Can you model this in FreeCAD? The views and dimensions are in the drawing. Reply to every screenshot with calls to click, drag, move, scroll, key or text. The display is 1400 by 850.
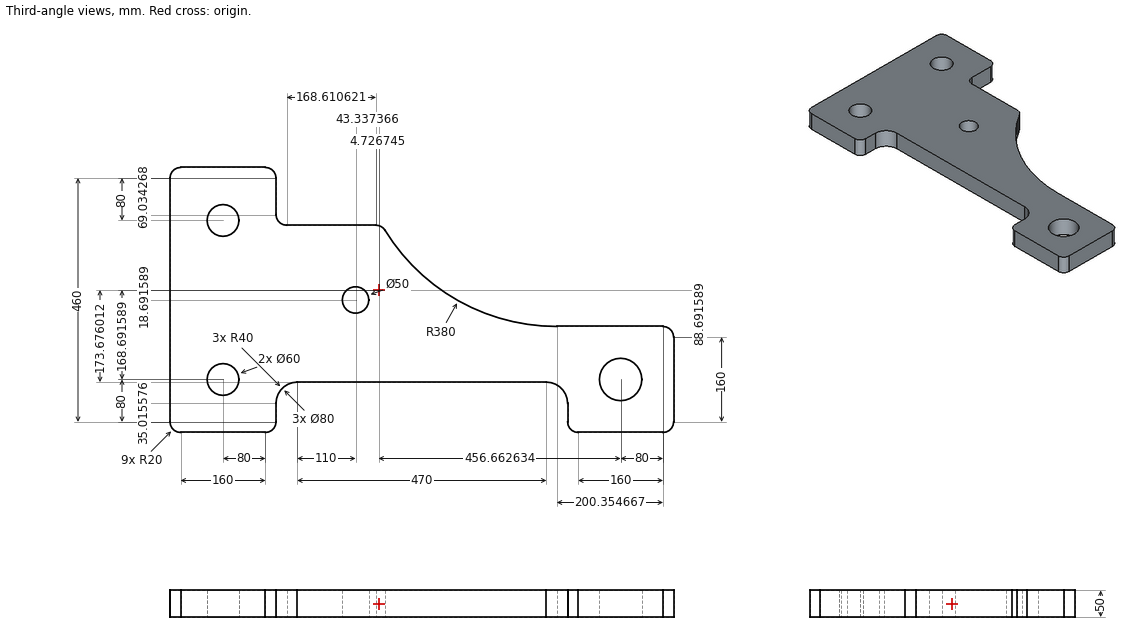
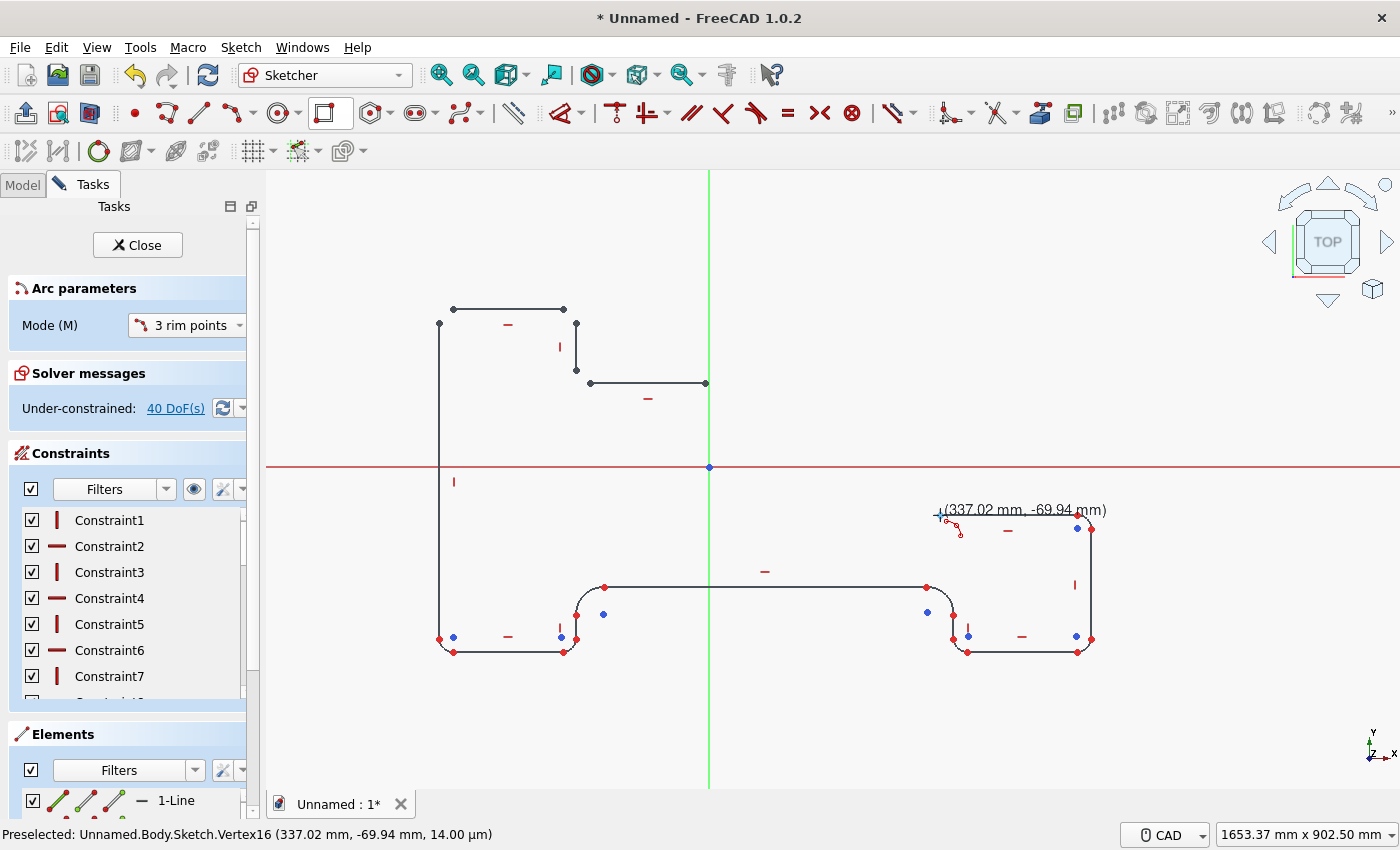
scroll(717, 390, up, 4)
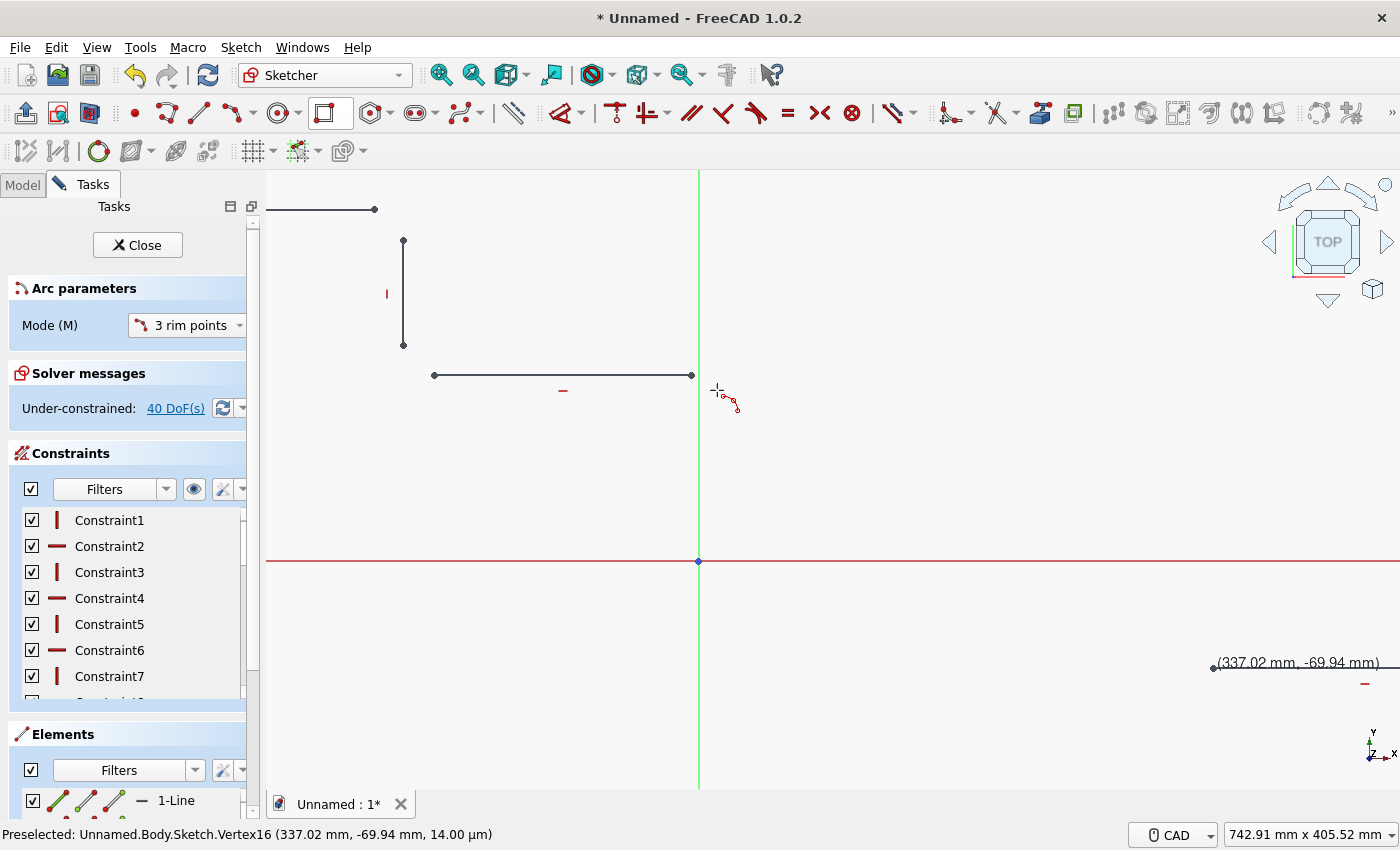
click(718, 389)
click(982, 619)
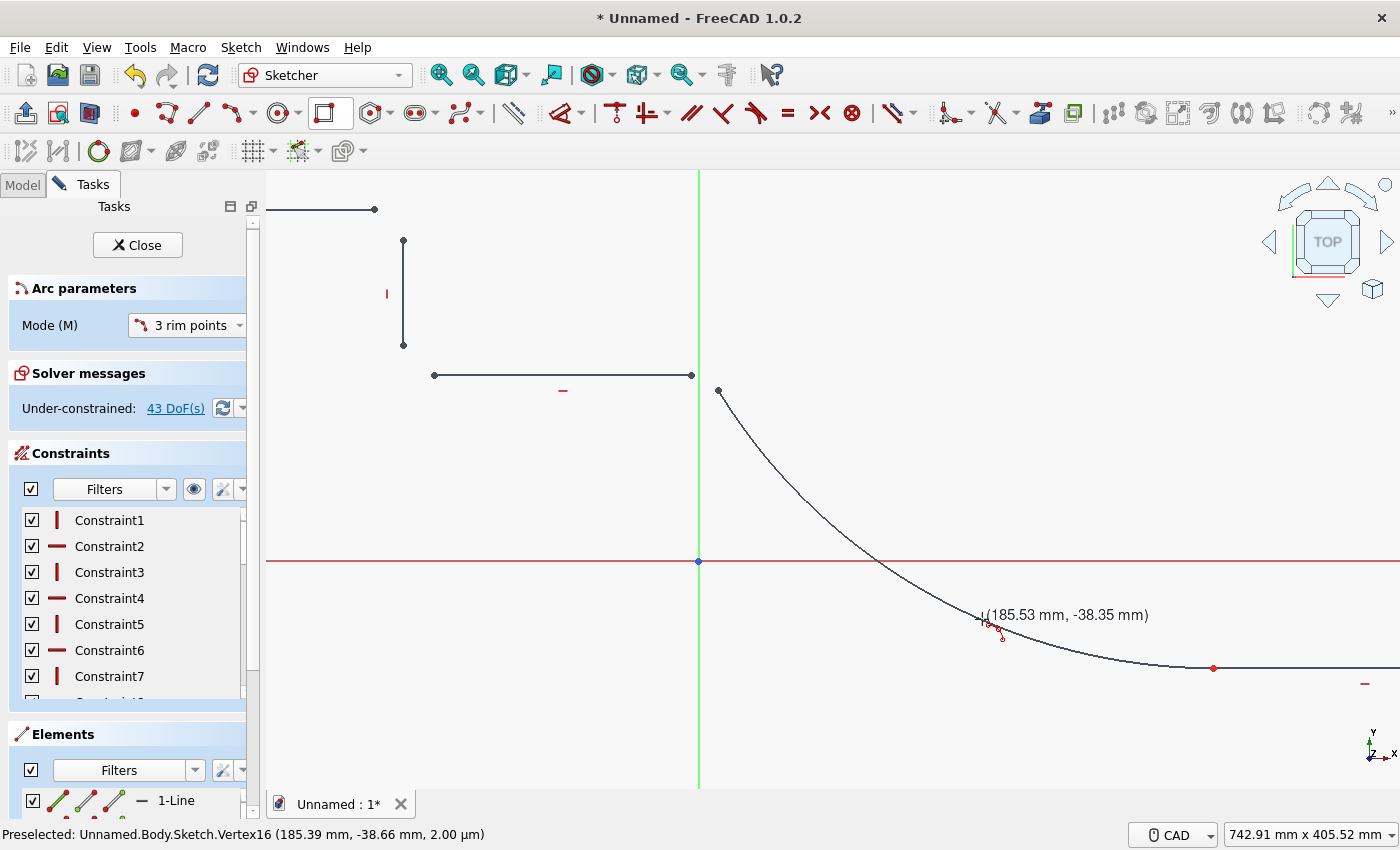
click(718, 390)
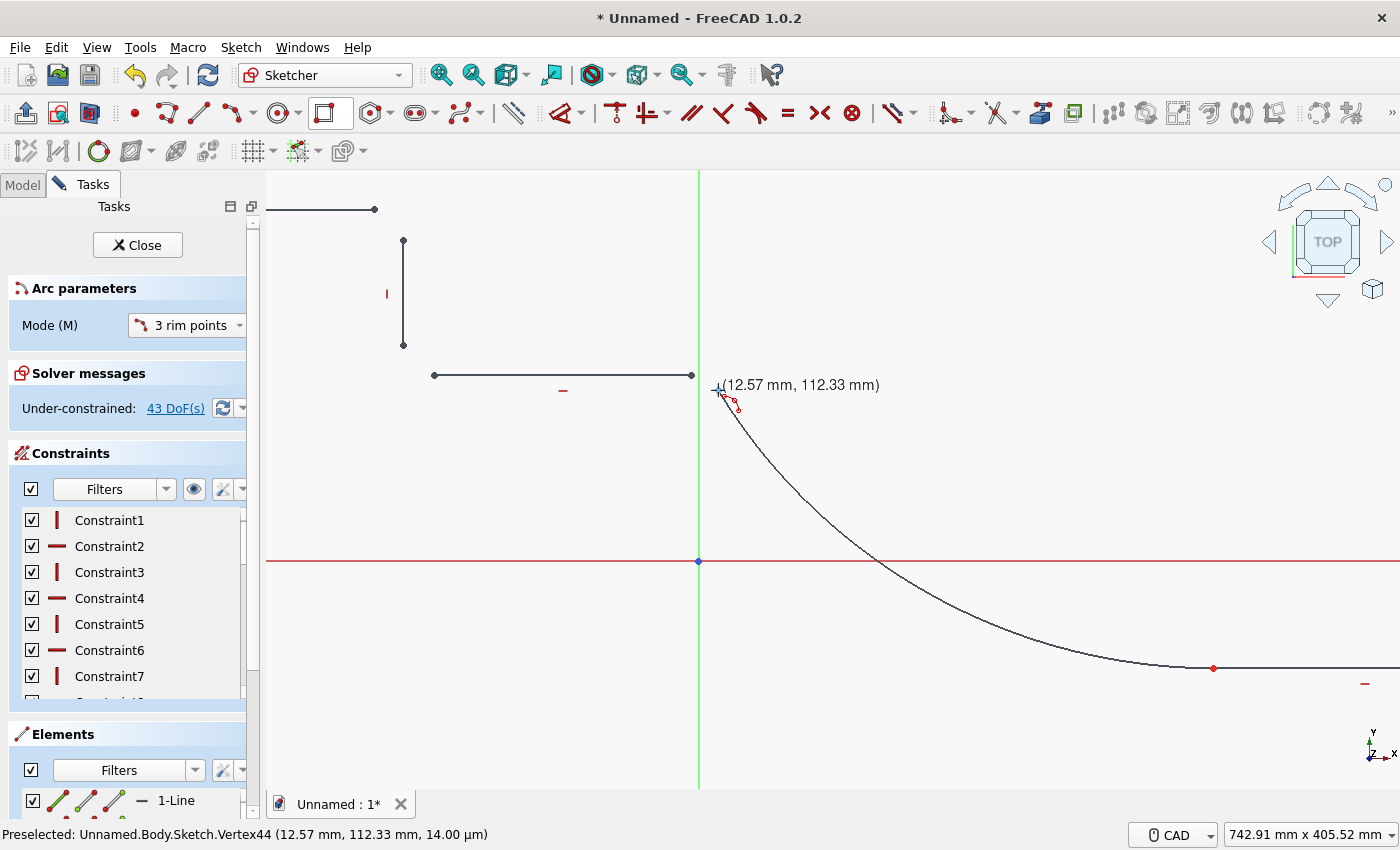
scroll(692, 375, up, 4)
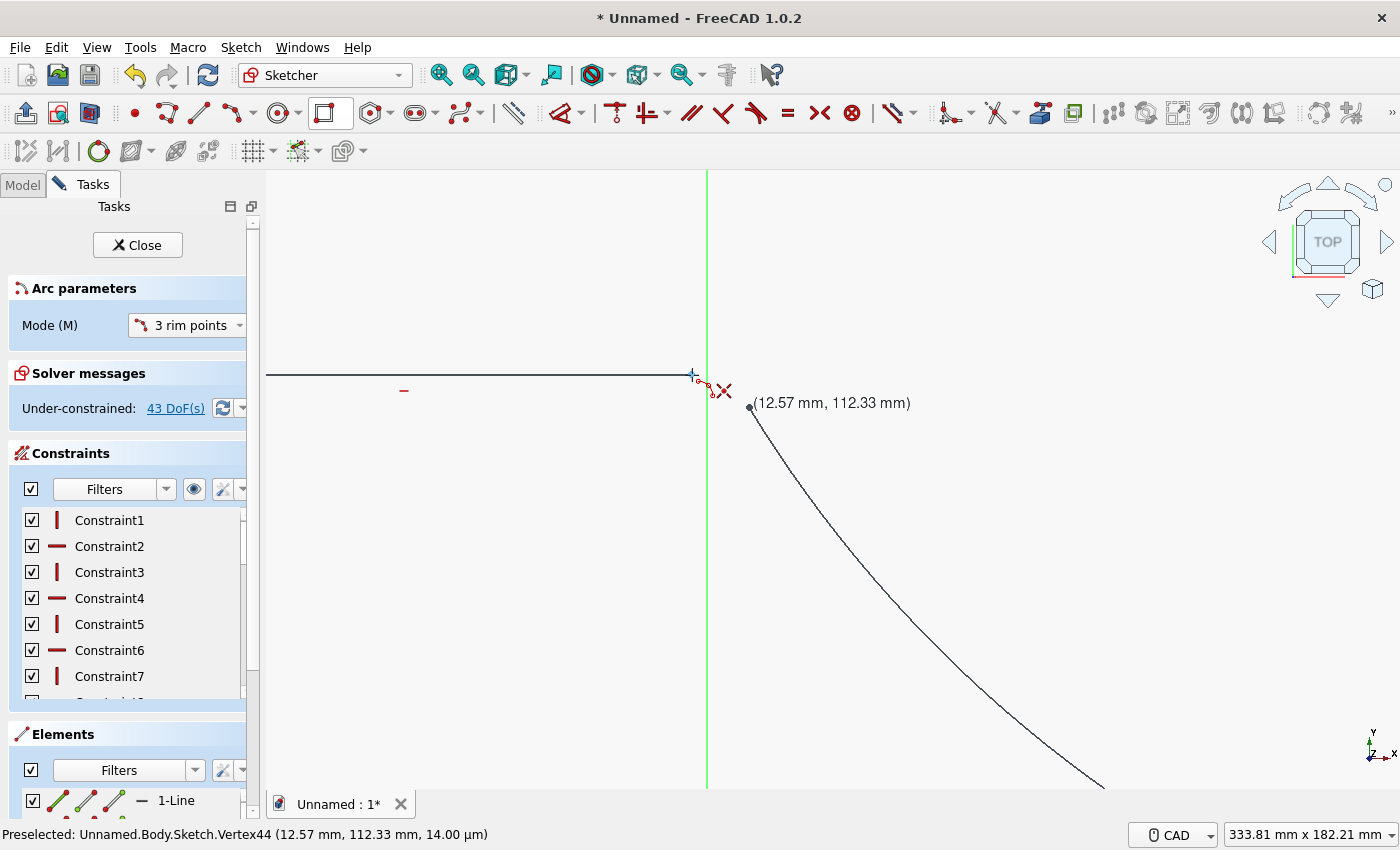
click(691, 375)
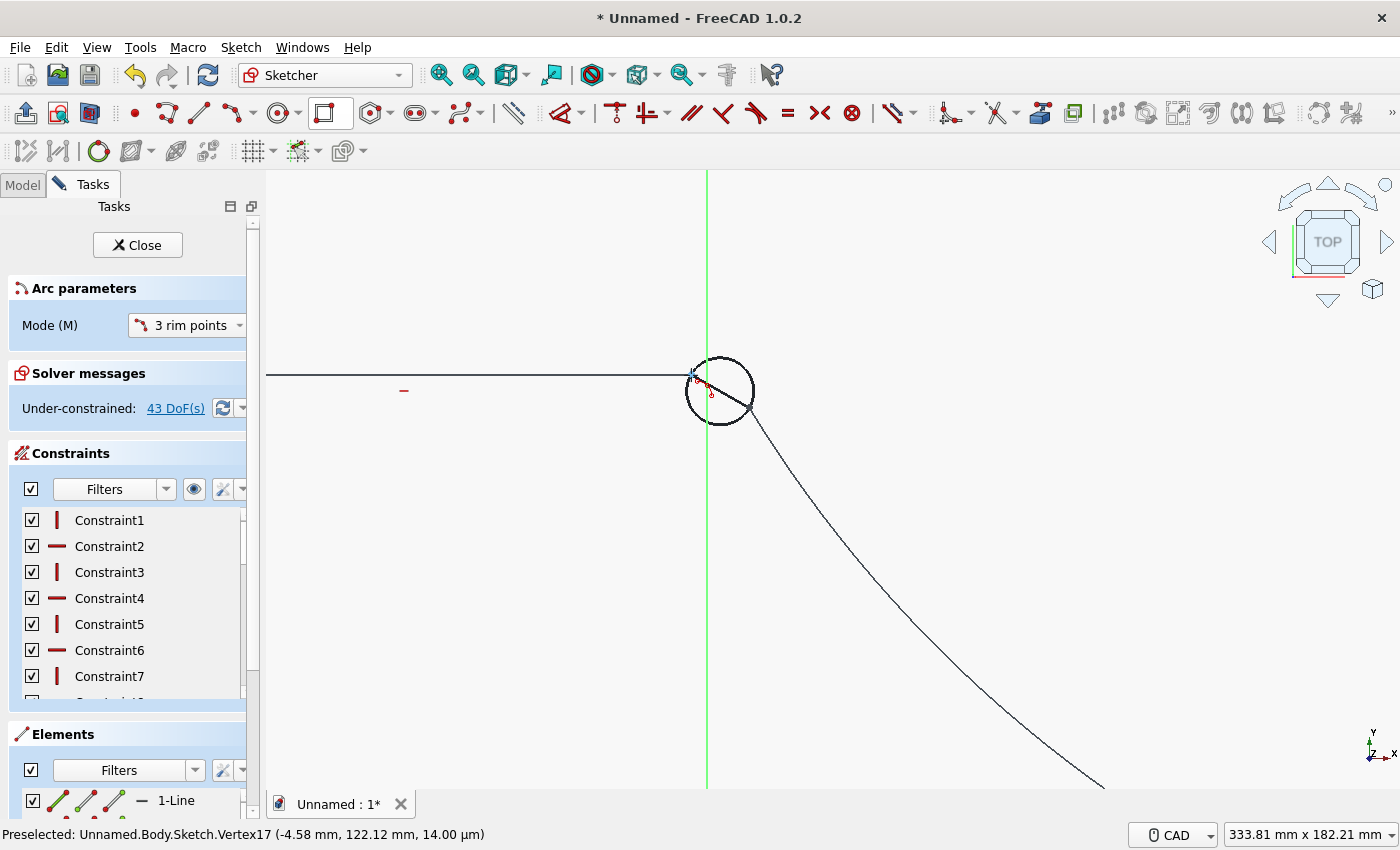
scroll(724, 383, up, 4)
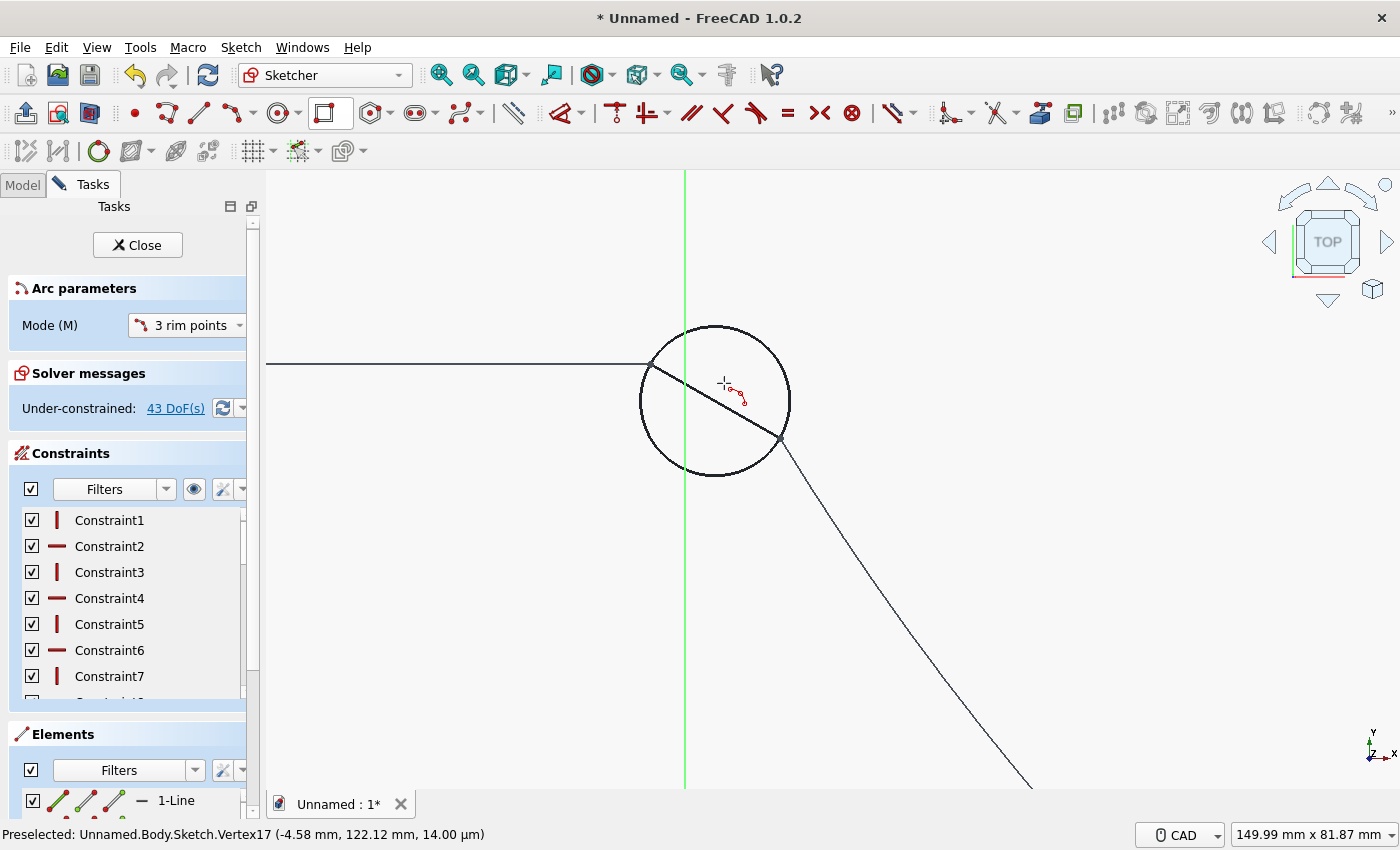
click(723, 382)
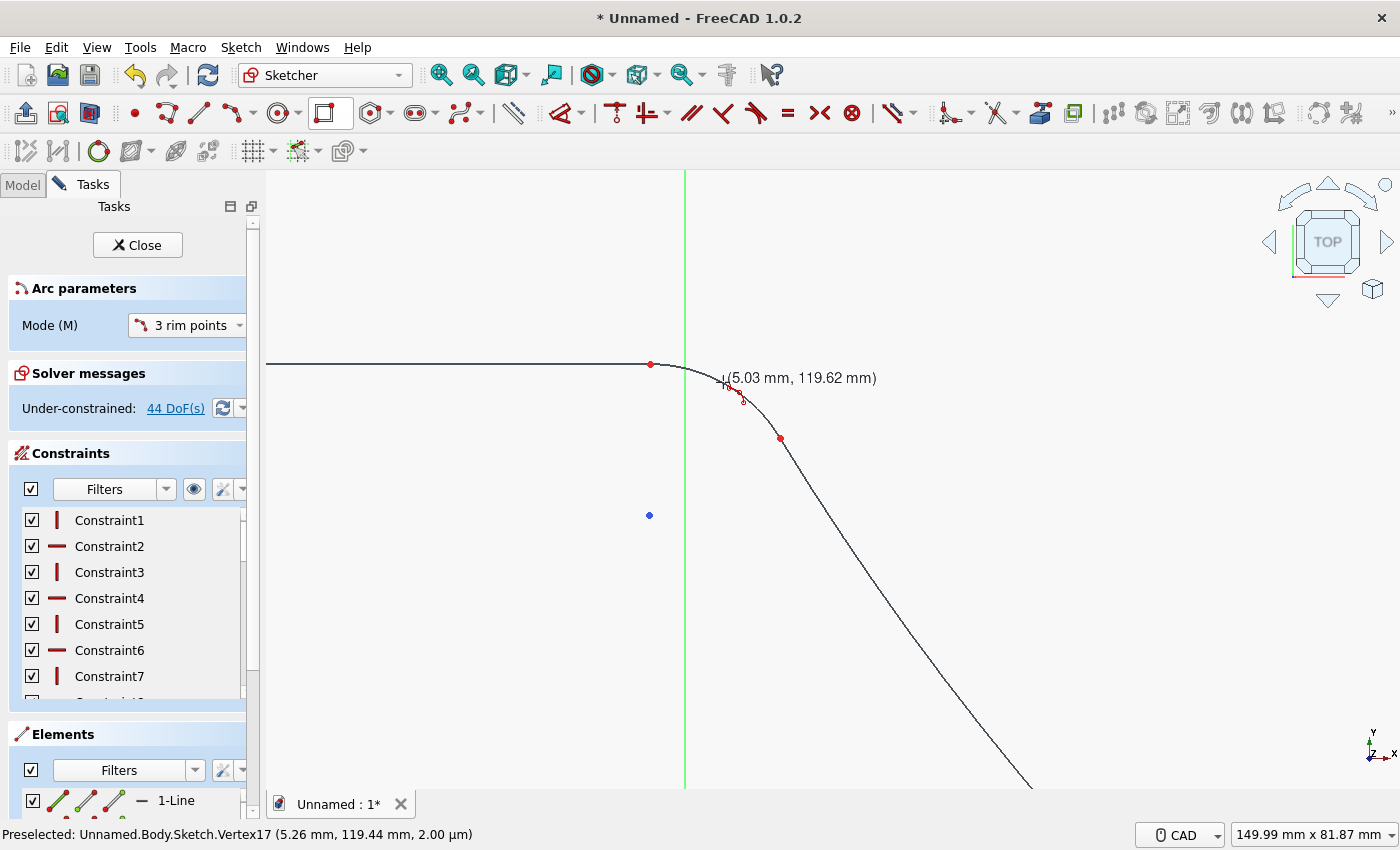
scroll(711, 385, down, 12)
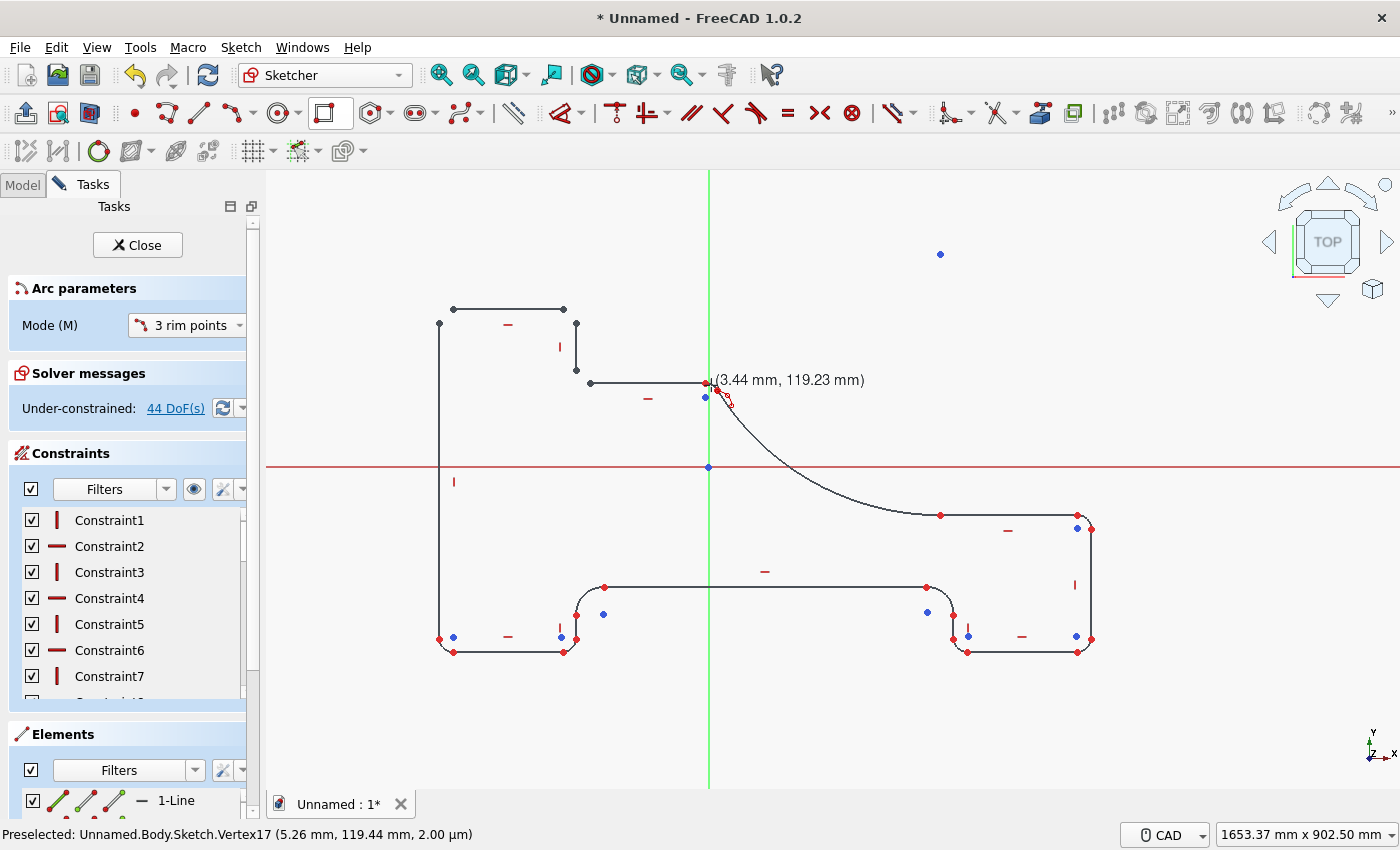
click(590, 383)
click(576, 370)